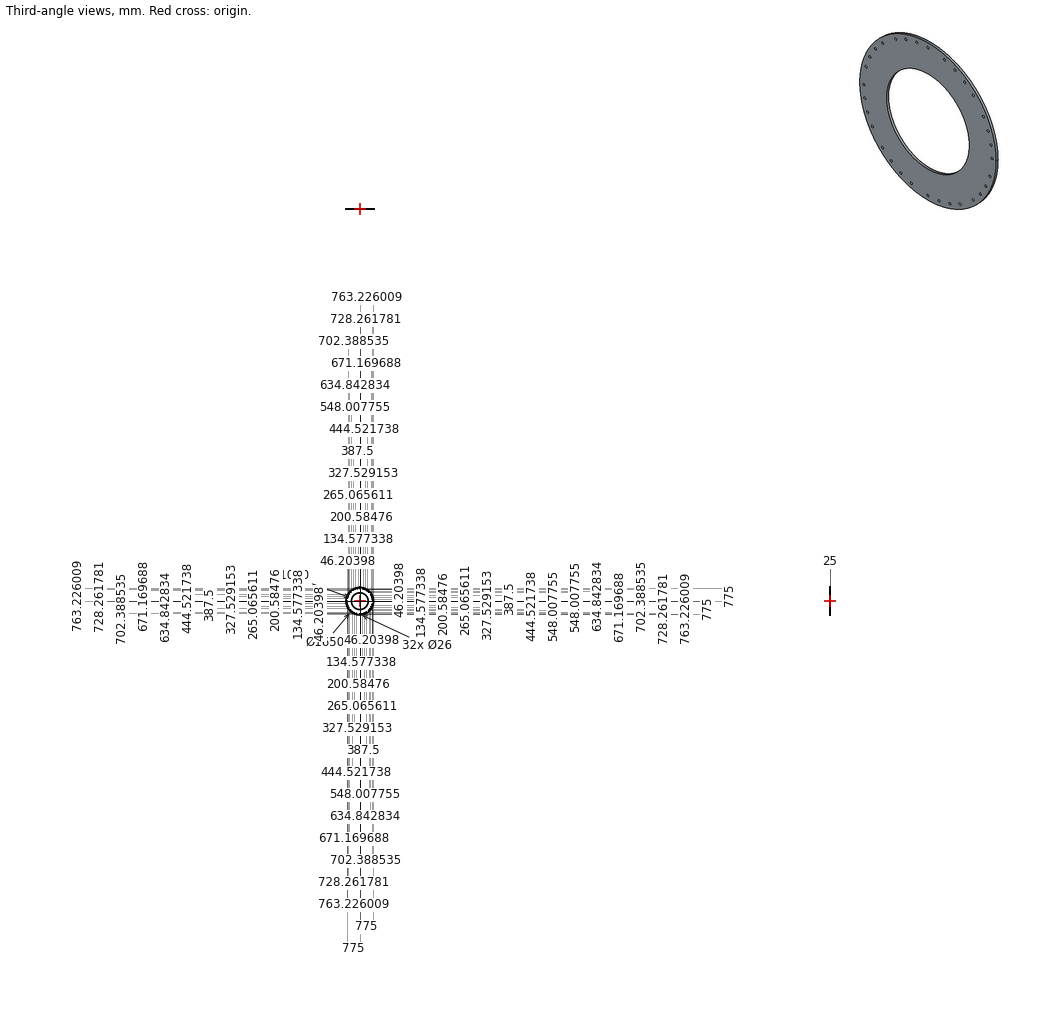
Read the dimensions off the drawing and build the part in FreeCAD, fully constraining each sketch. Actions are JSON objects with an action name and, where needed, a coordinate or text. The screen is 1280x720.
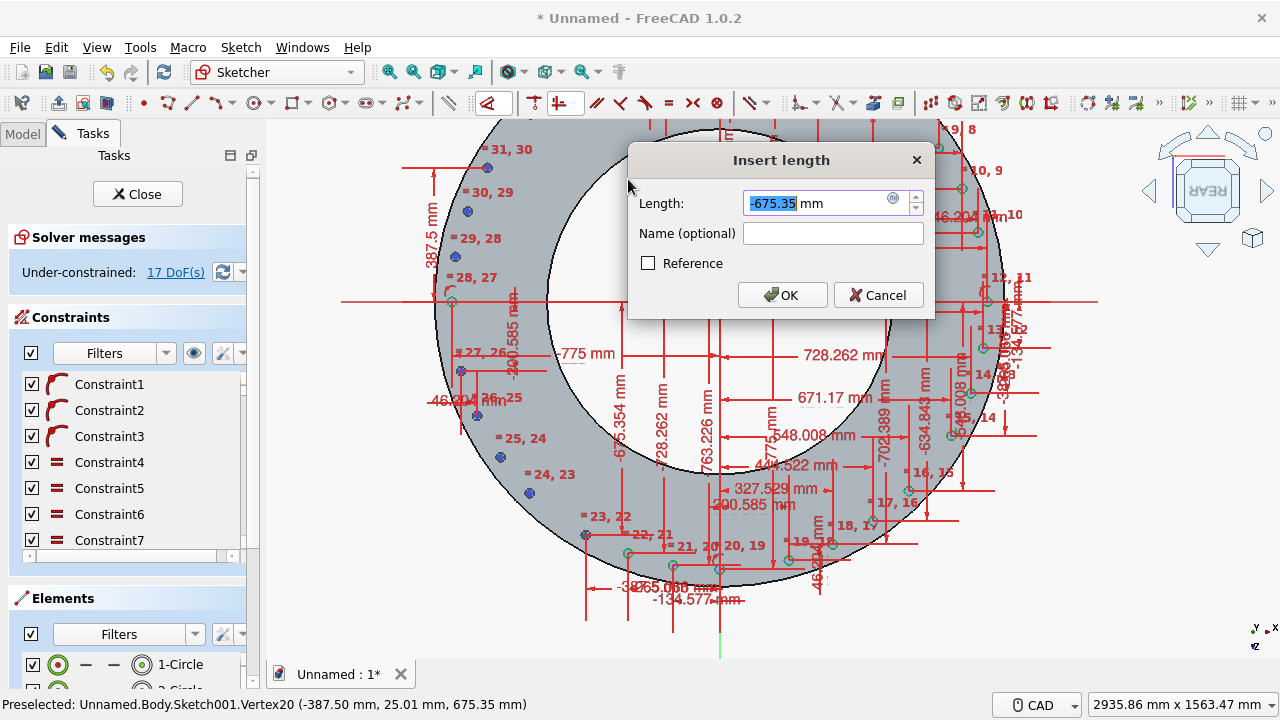
{"action": "type", "text": "-671.169688"}
{"action": "key", "text": "Return"}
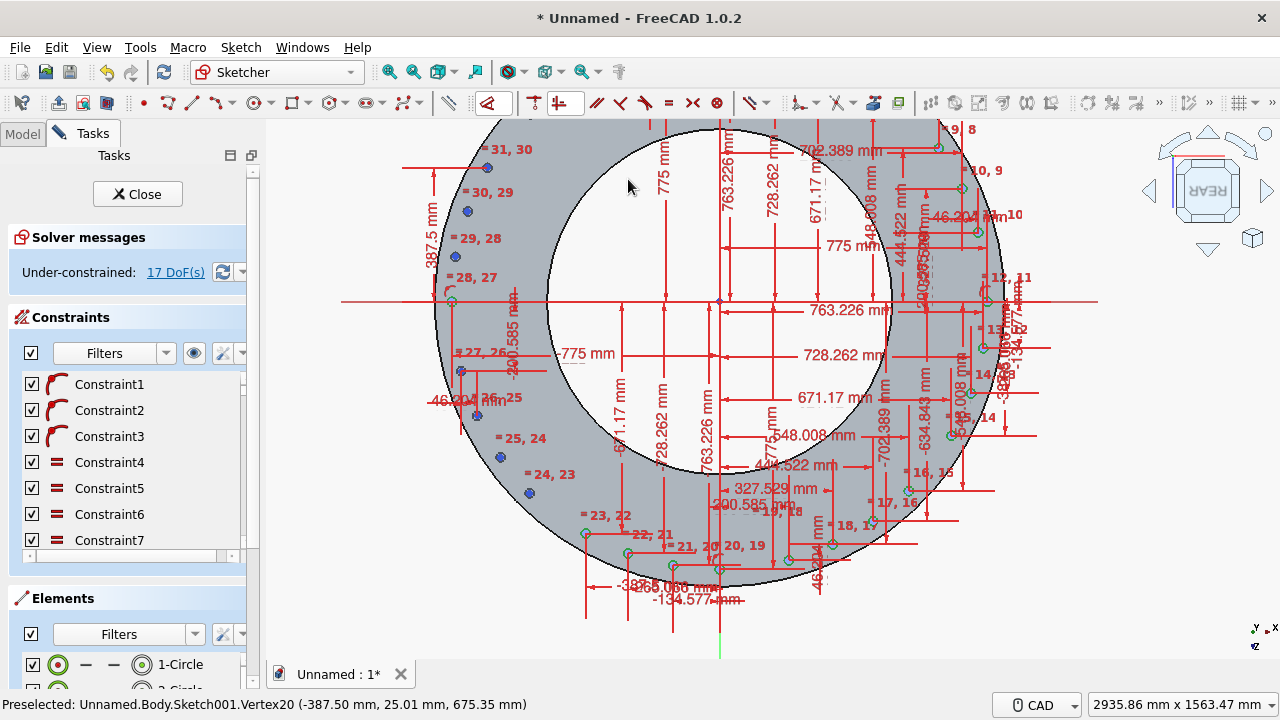
{"action": "left_click", "coordinate": [530, 493]}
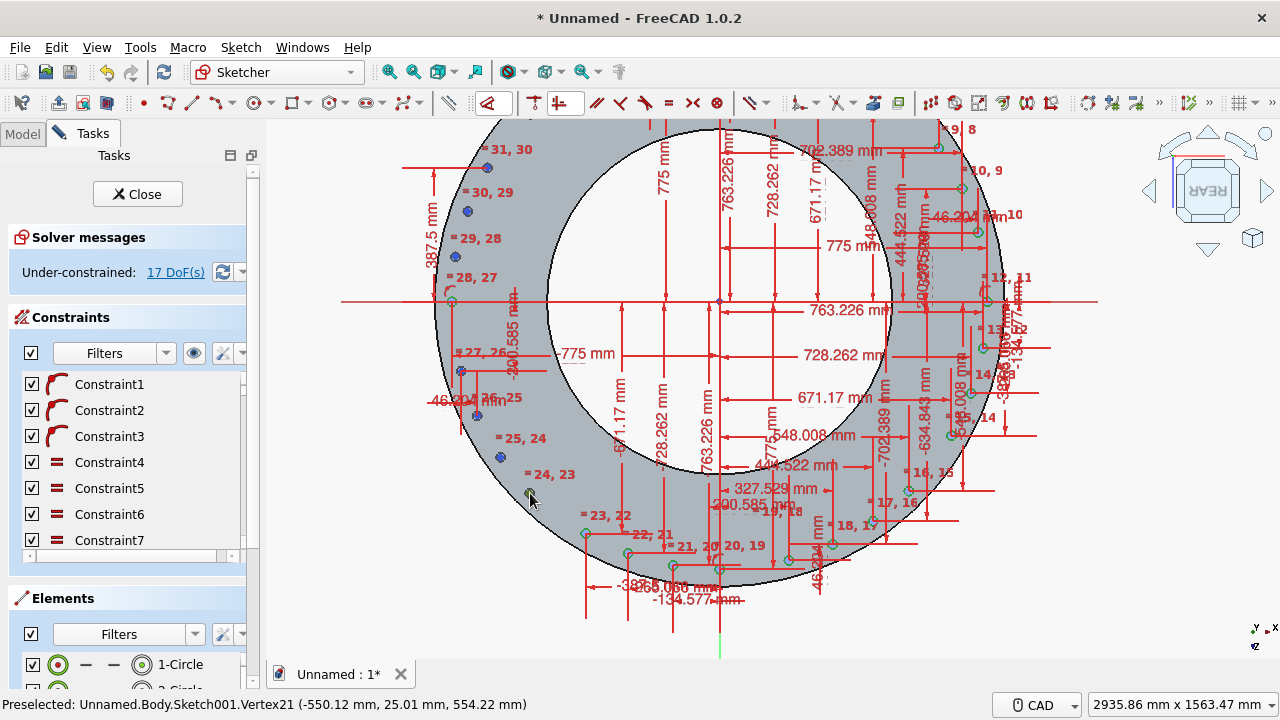
{"action": "key", "text": "l"}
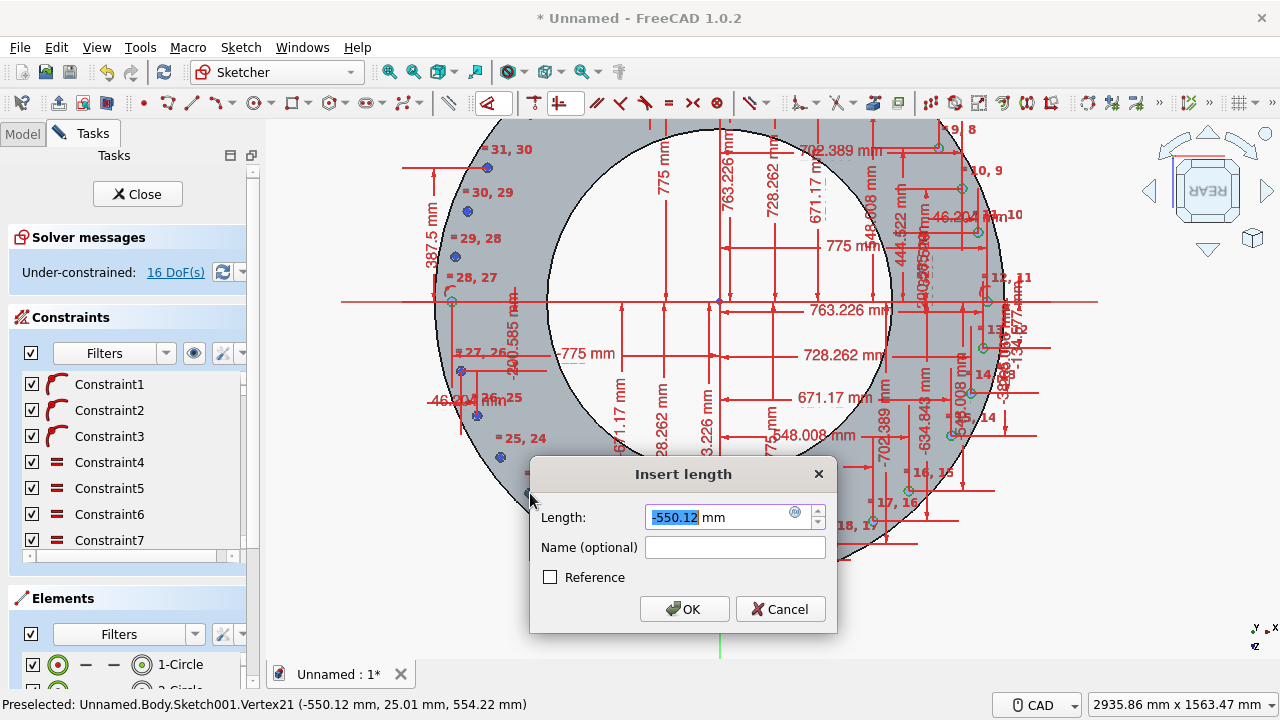
{"action": "type", "text": "-548.007755"}
{"action": "key", "text": "Return"}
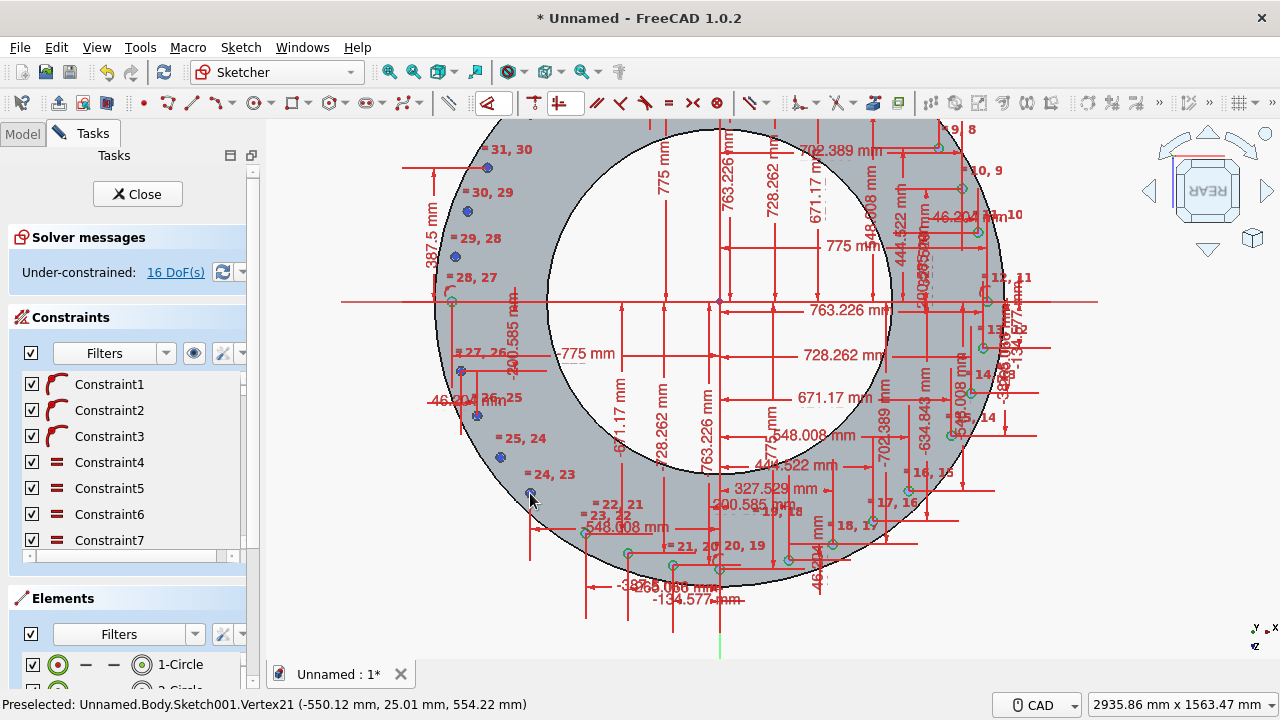
{"action": "left_click", "coordinate": [530, 493]}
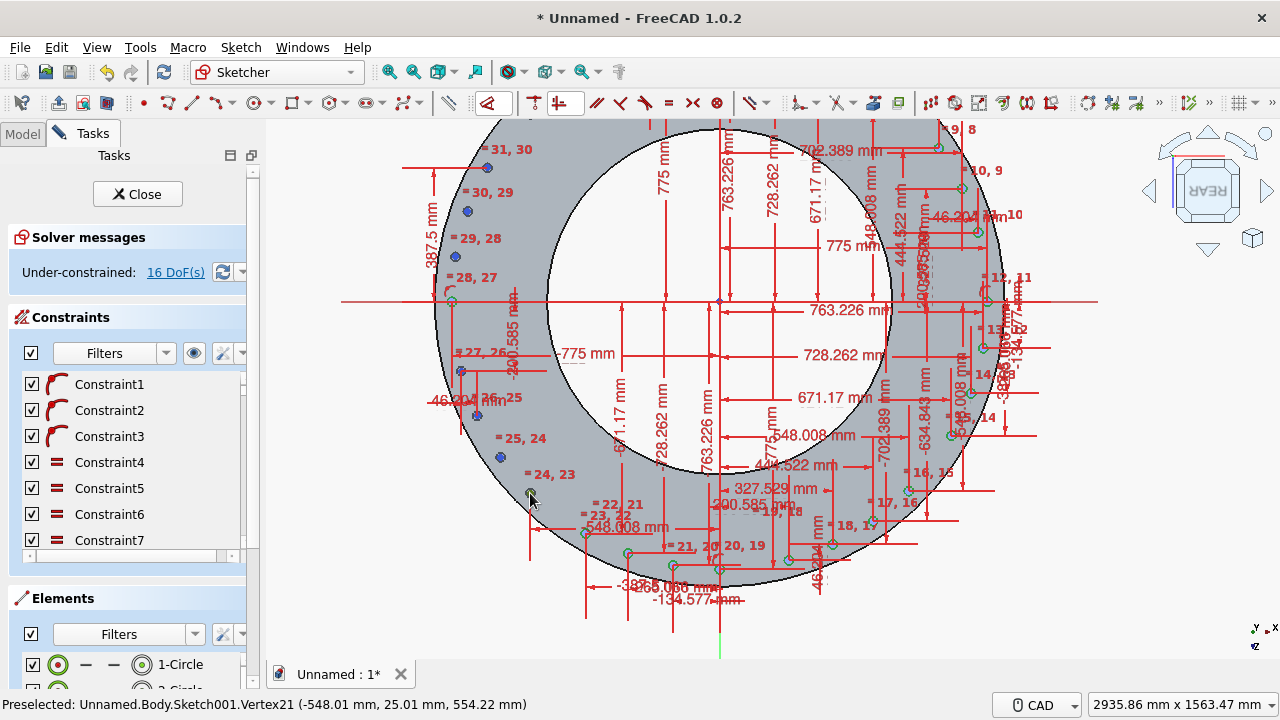
{"action": "key", "text": "i"}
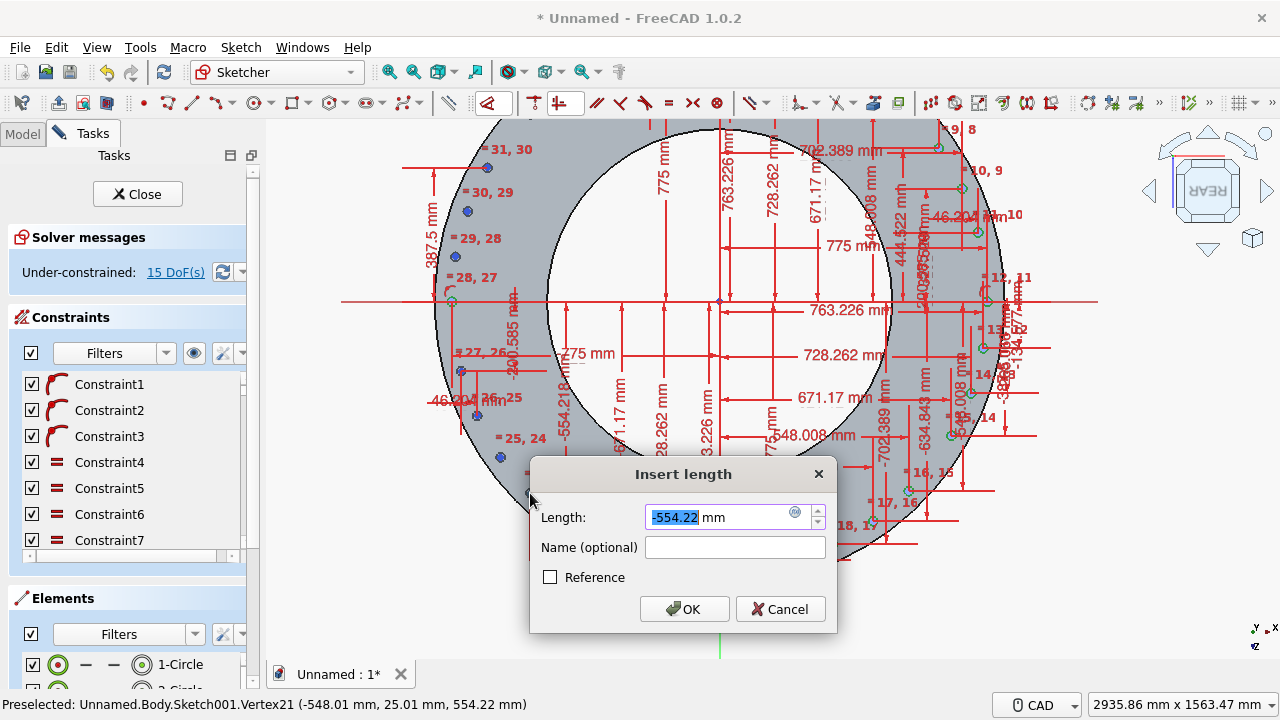
{"action": "type", "text": "-548.007755"}
{"action": "key", "text": "Return"}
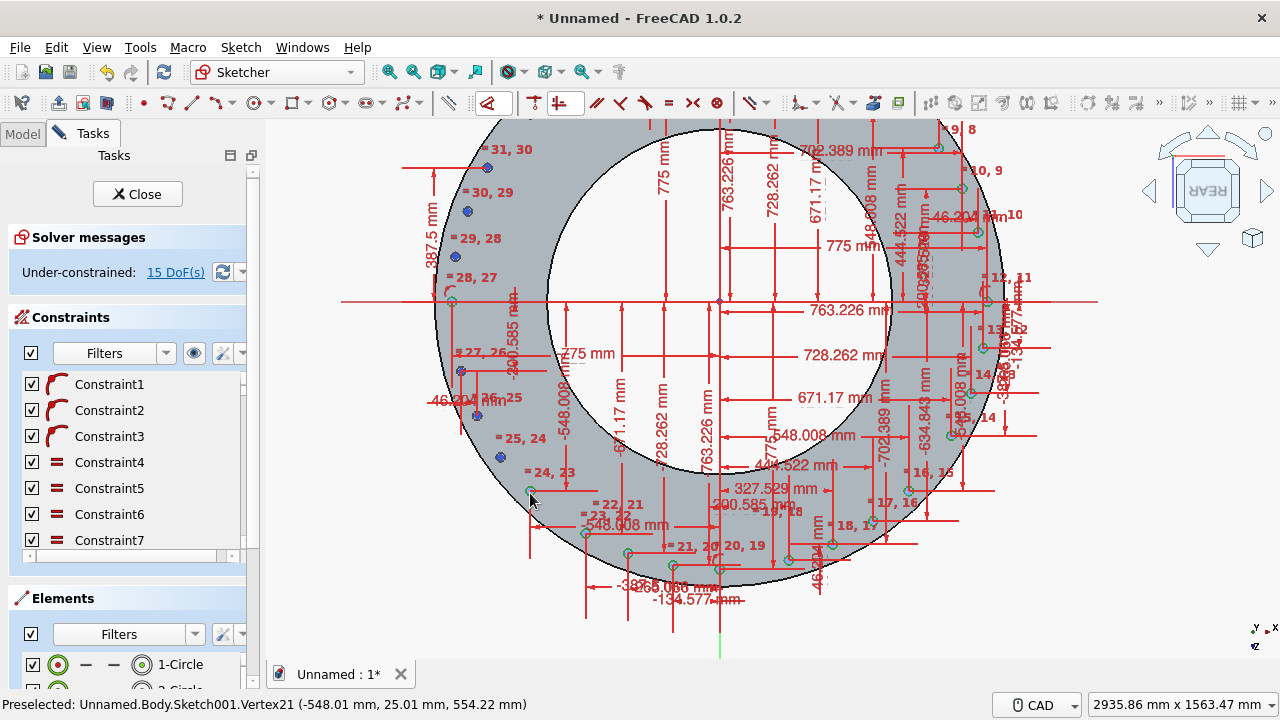
{"action": "left_click", "coordinate": [501, 457]}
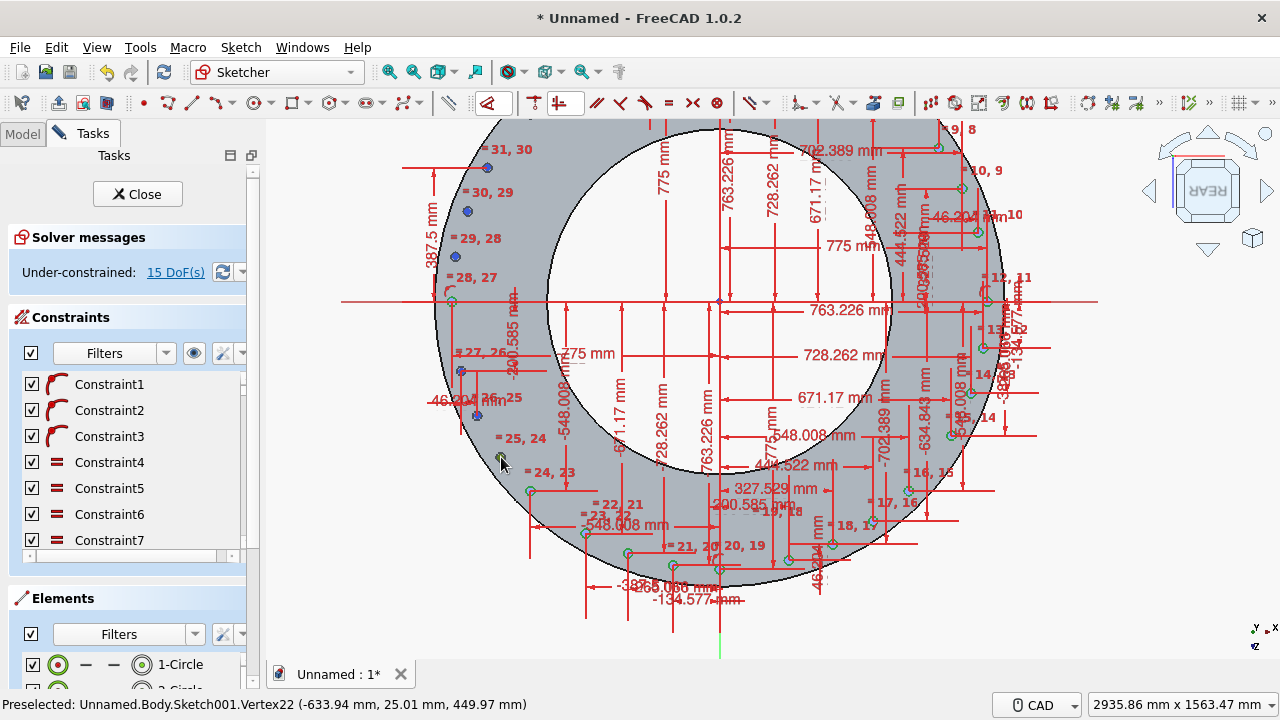
{"action": "key", "text": "l"}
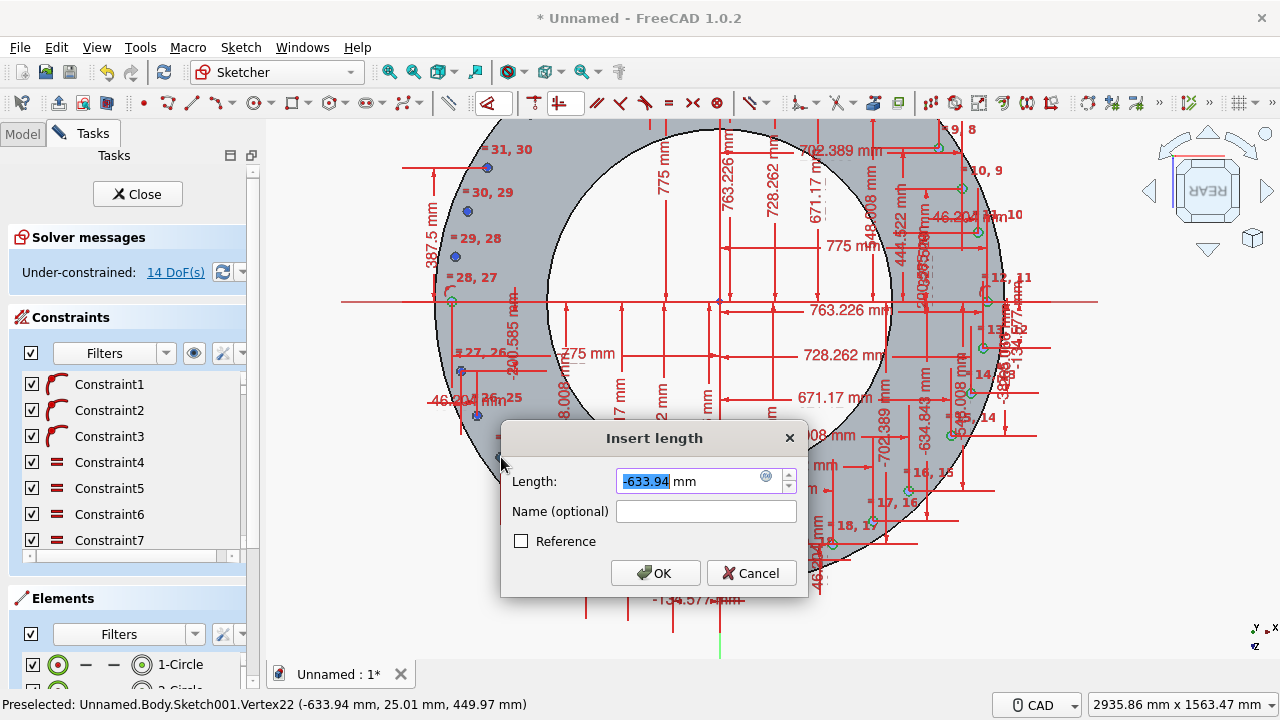
{"action": "type", "text": "-634.842834"}
{"action": "key", "text": "Return"}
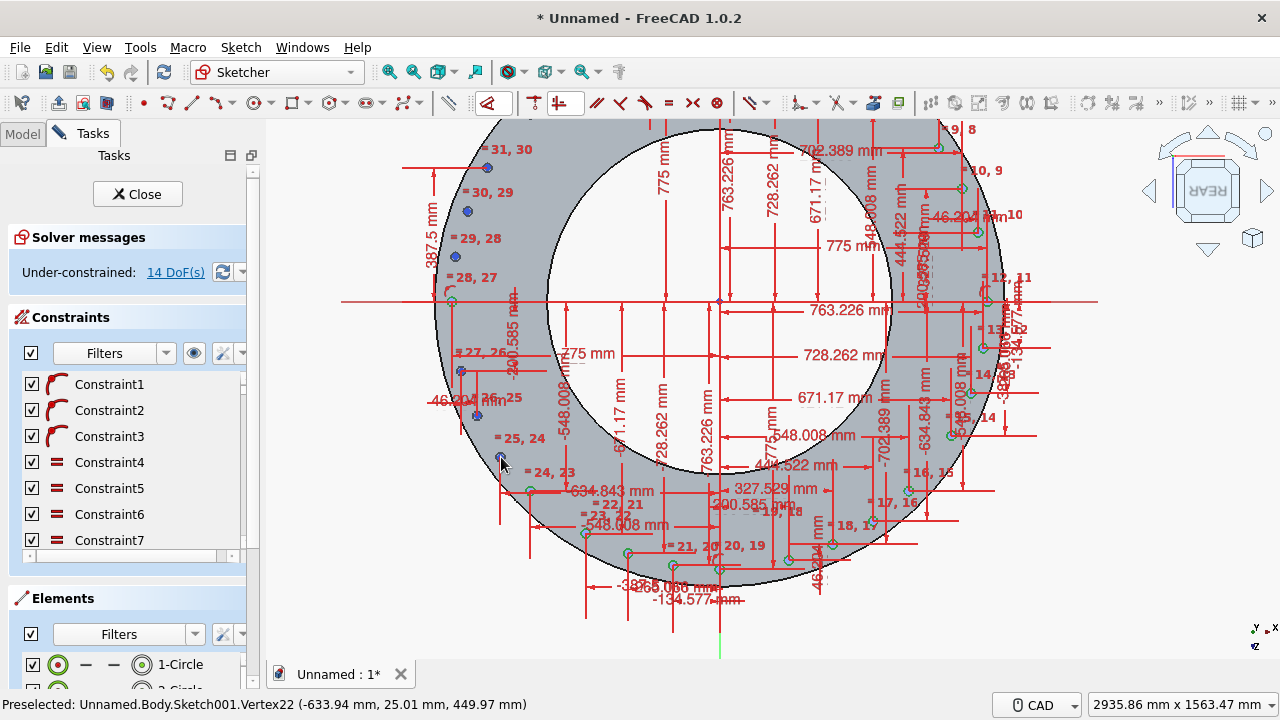
{"action": "left_click", "coordinate": [500, 457]}